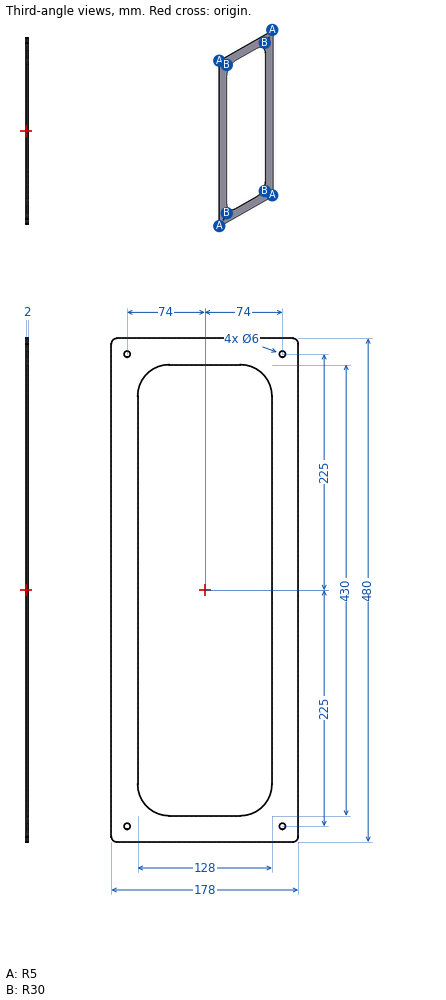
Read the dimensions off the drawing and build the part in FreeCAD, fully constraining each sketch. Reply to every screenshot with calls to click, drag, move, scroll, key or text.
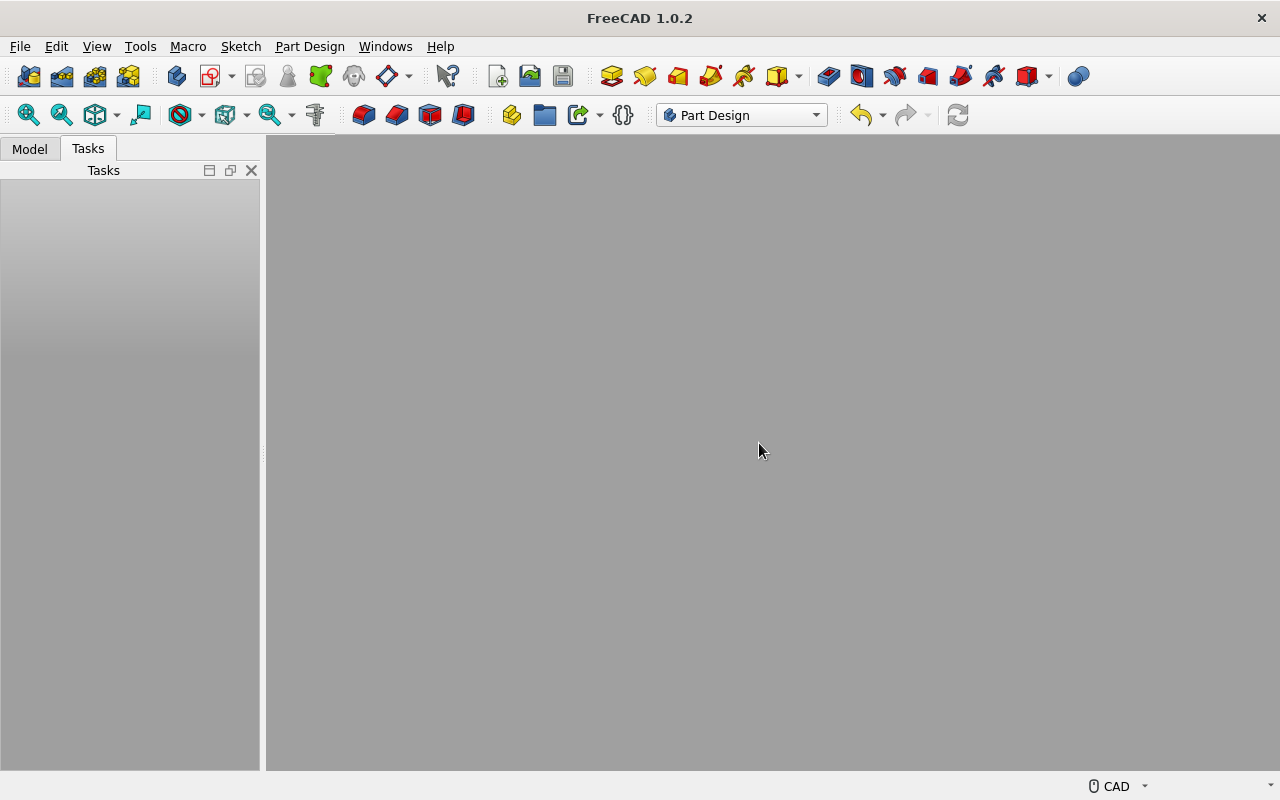
click(497, 76)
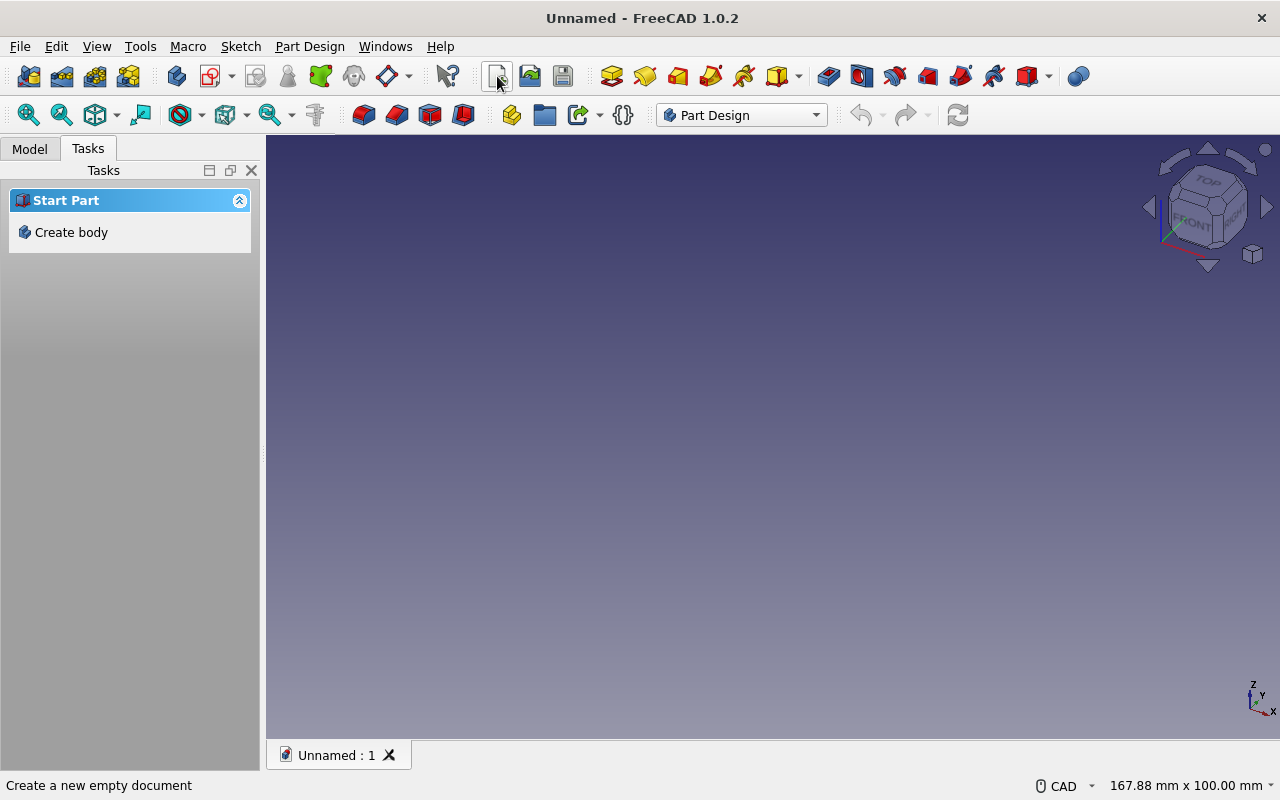
click(210, 76)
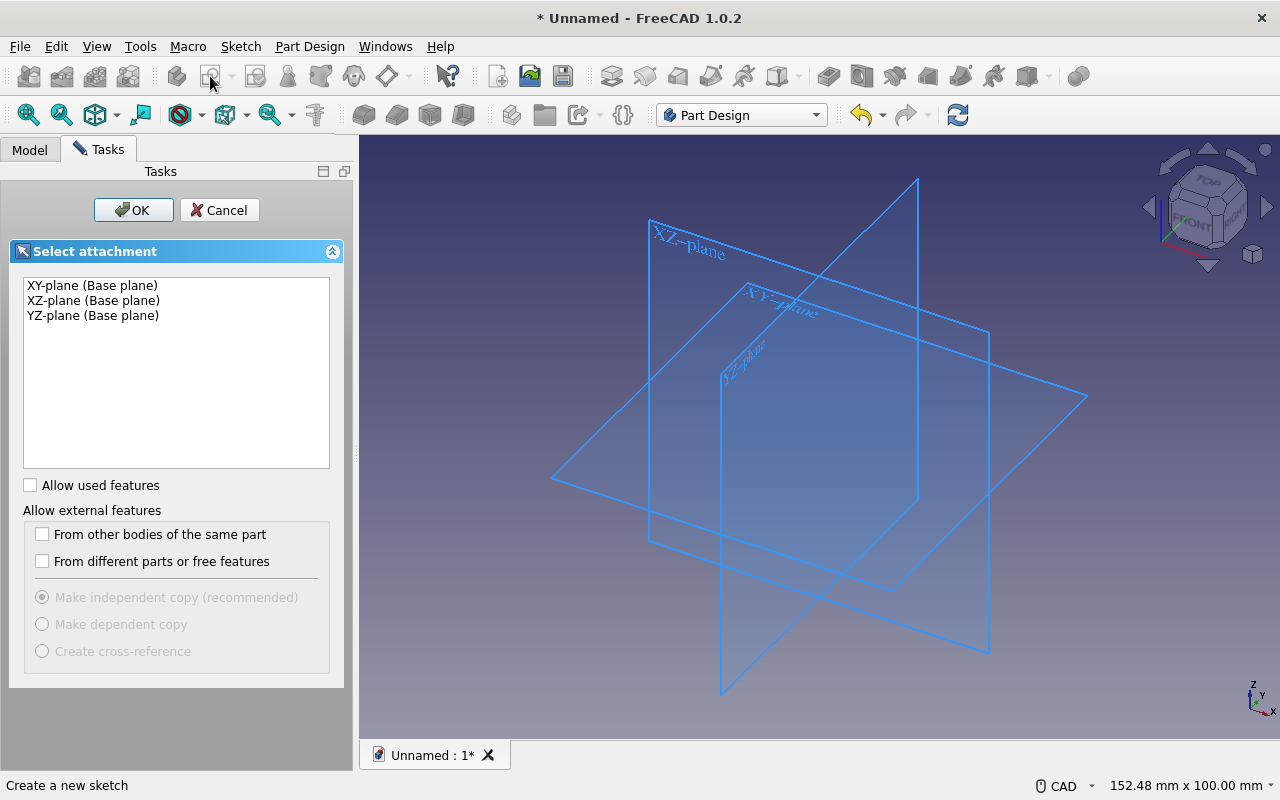
click(84, 316)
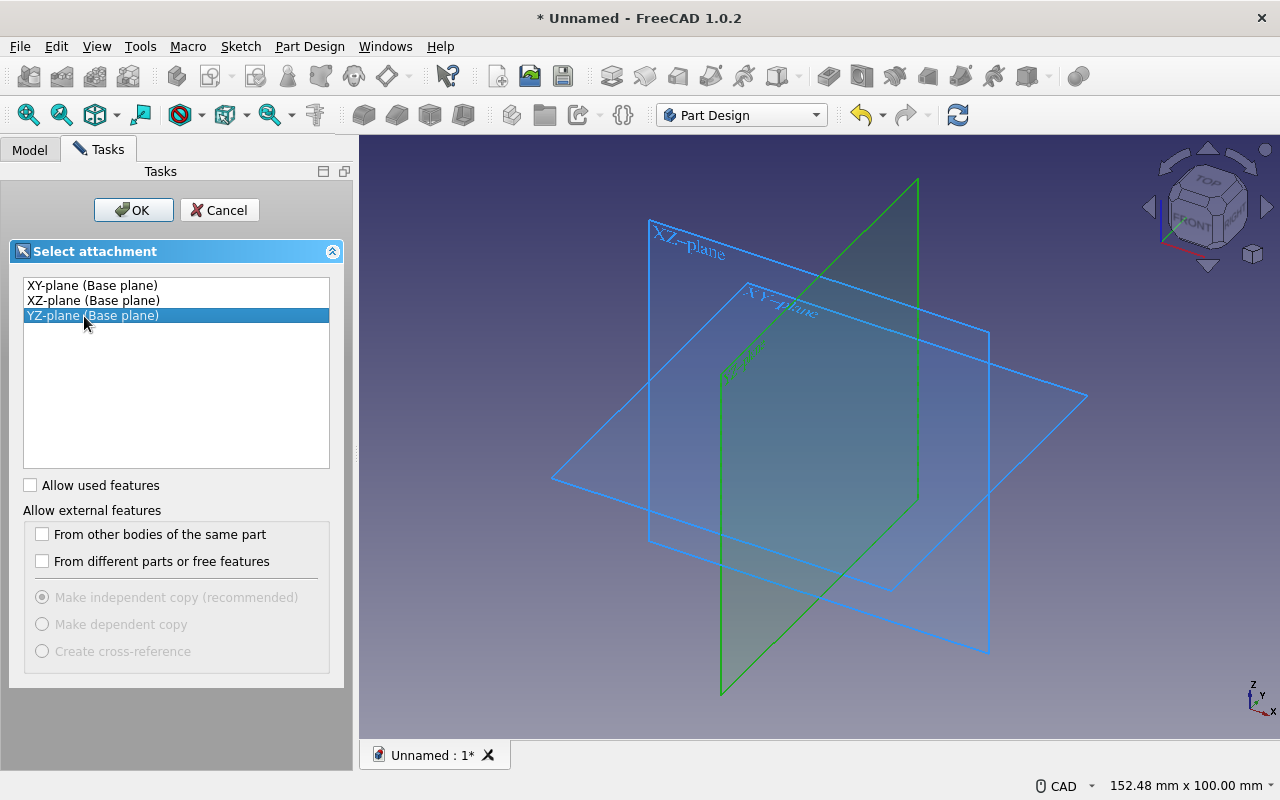
click(134, 210)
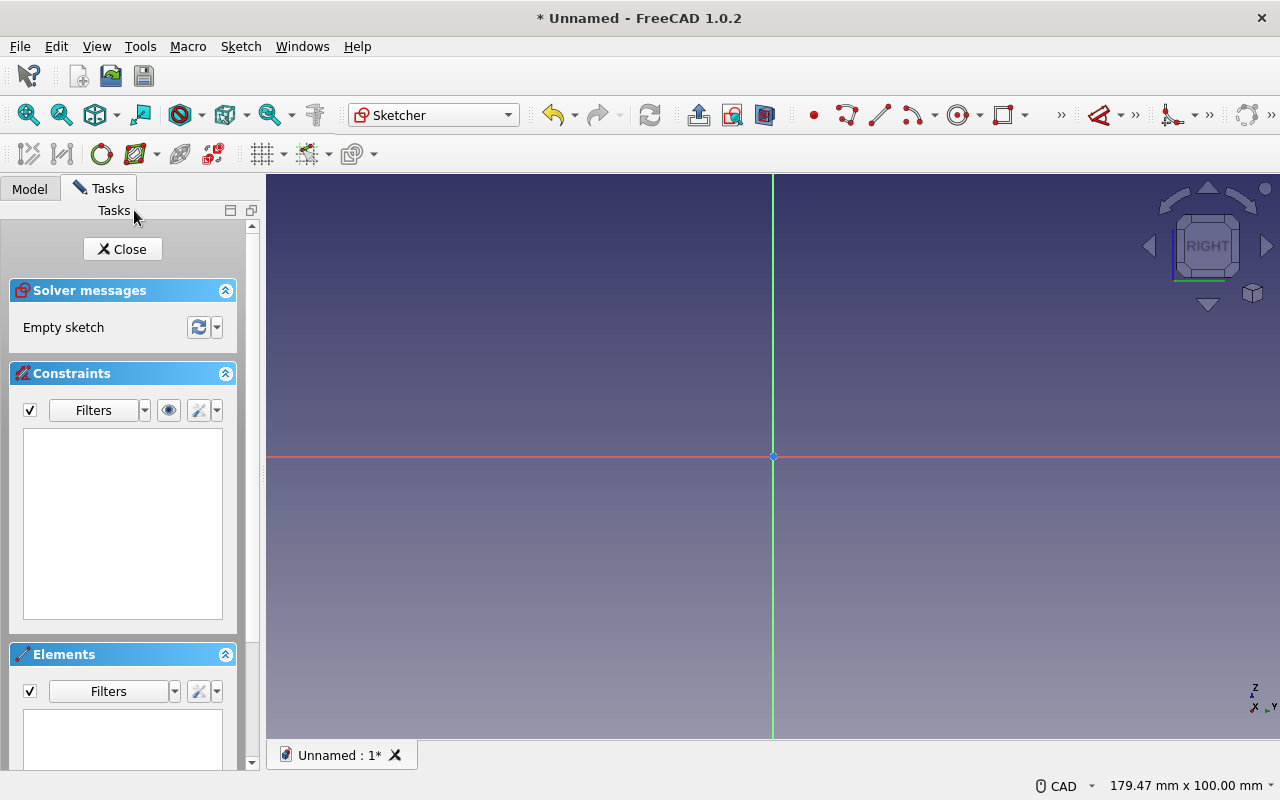
scroll(694, 457, down, 10)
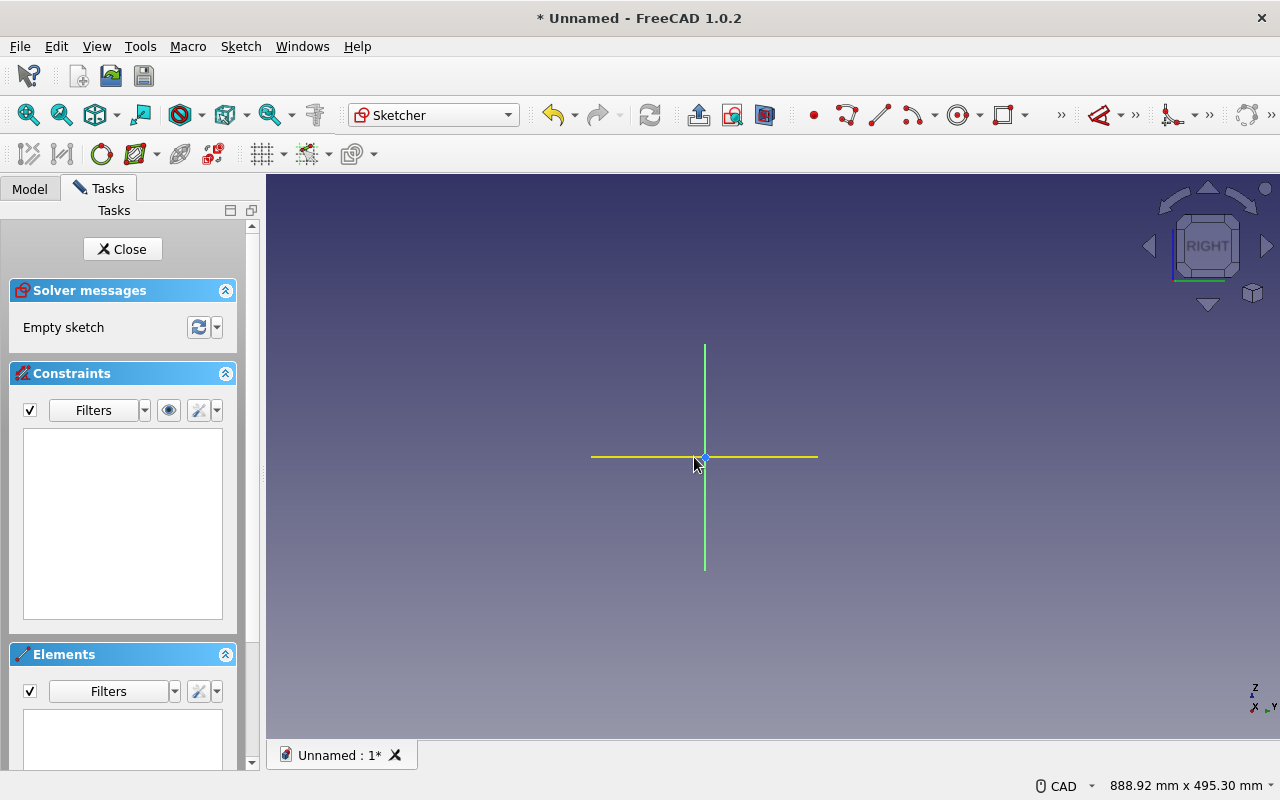
key(g)
key(v)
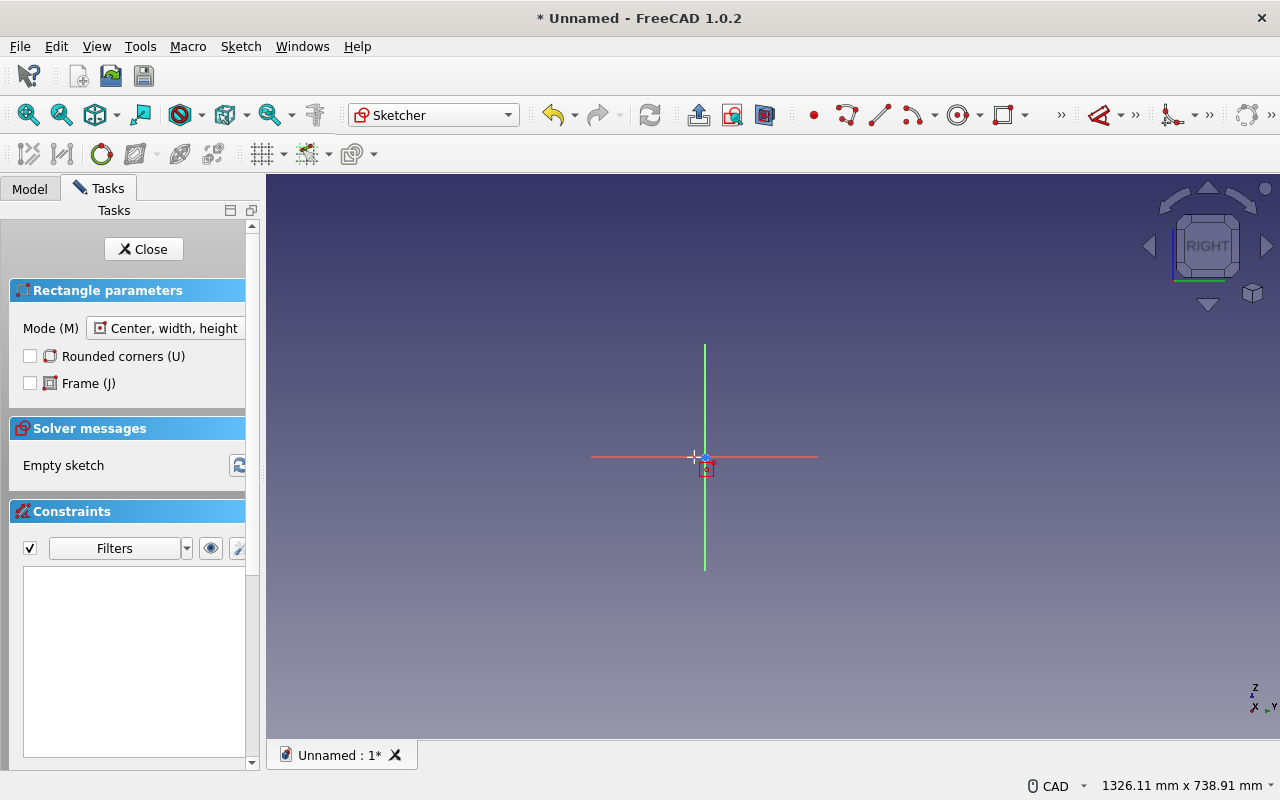
click(705, 457)
move(773, 274)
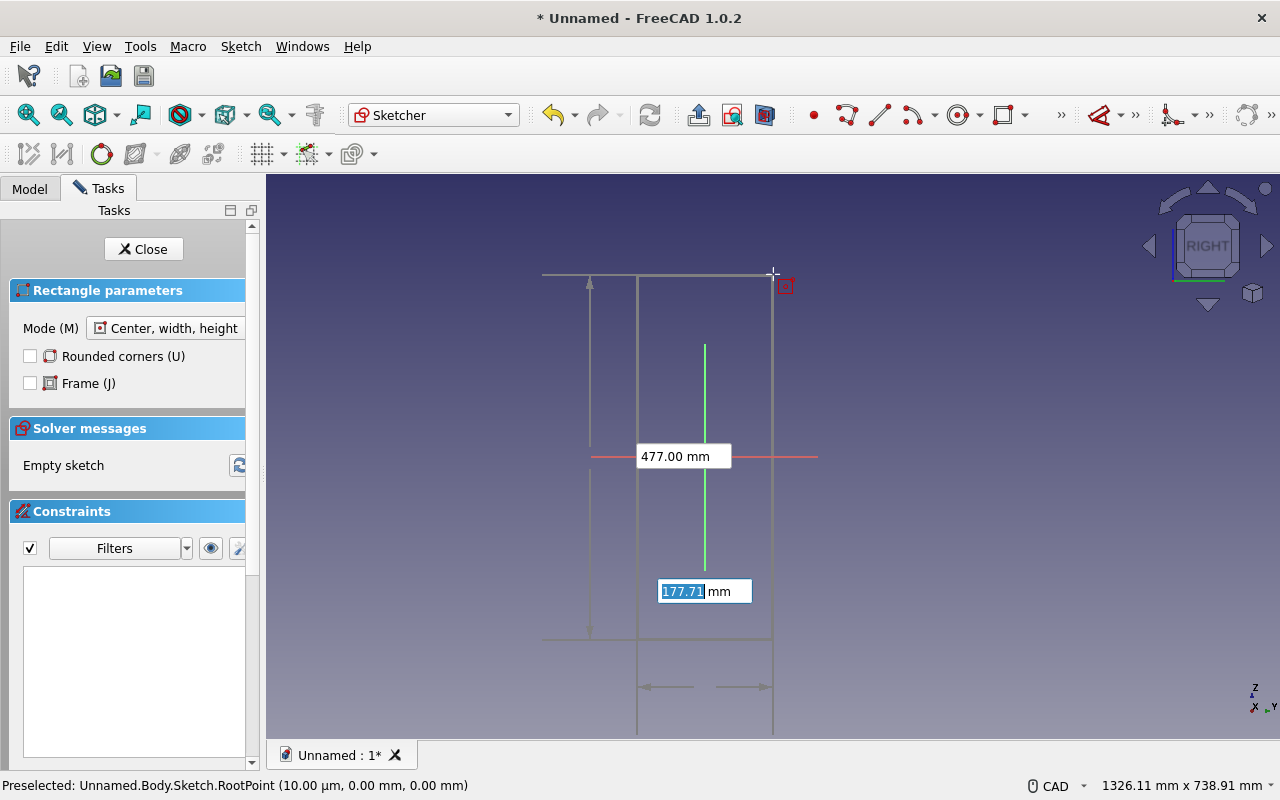
text(178)
key(Tab)
text(480)
key(Return)
key(Escape)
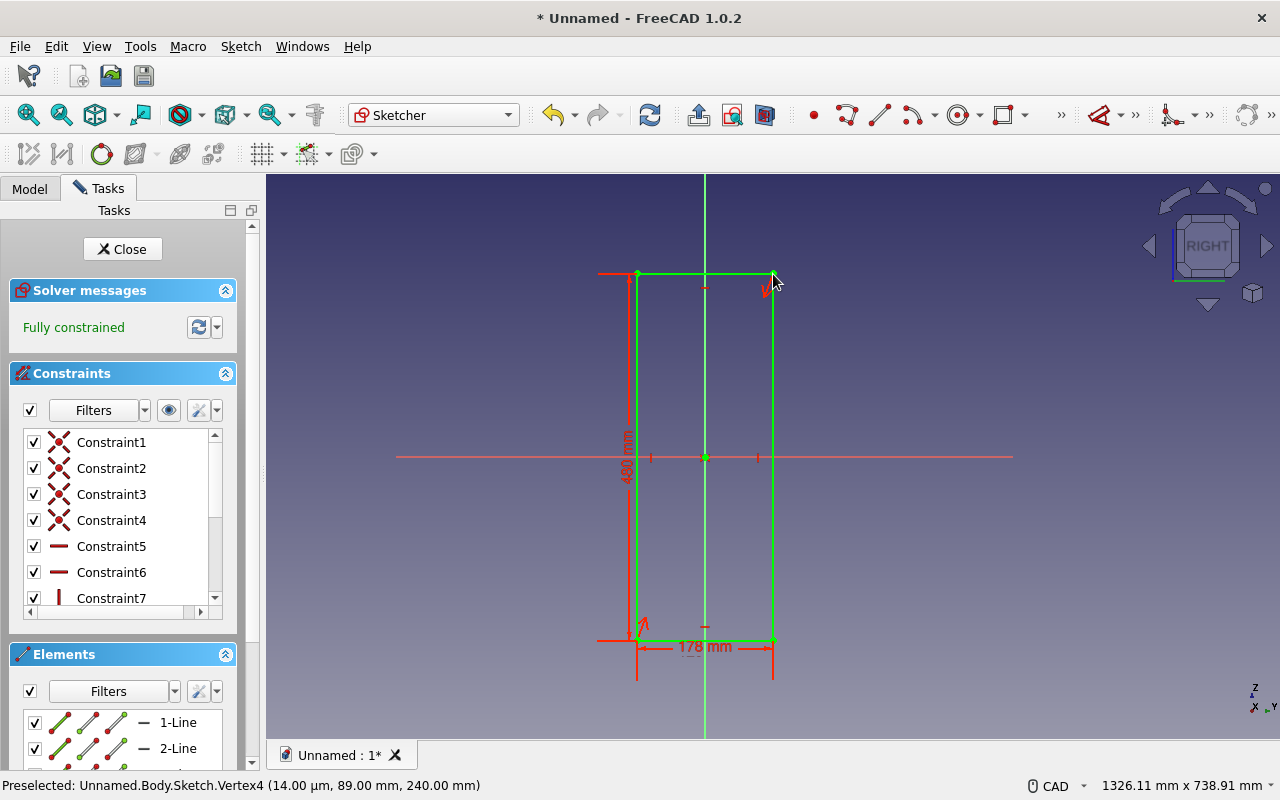
click(123, 249)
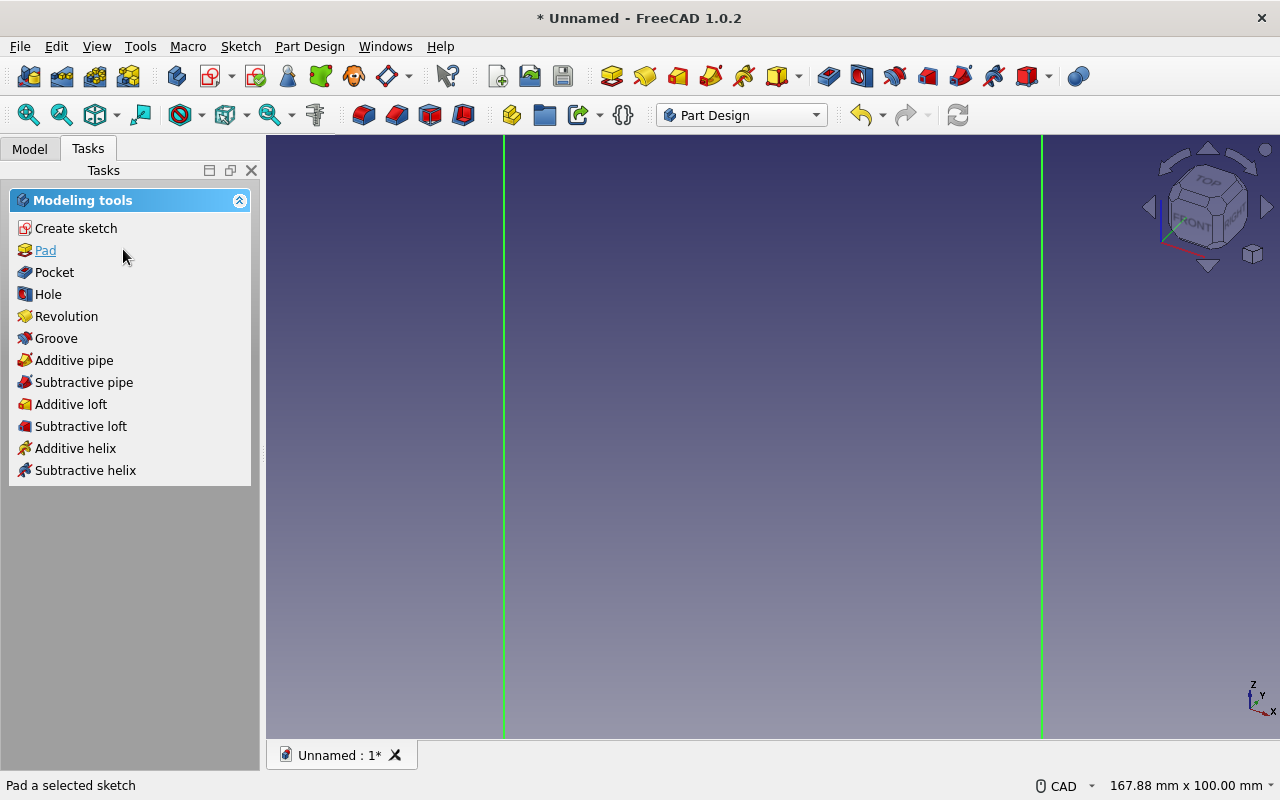
click(612, 76)